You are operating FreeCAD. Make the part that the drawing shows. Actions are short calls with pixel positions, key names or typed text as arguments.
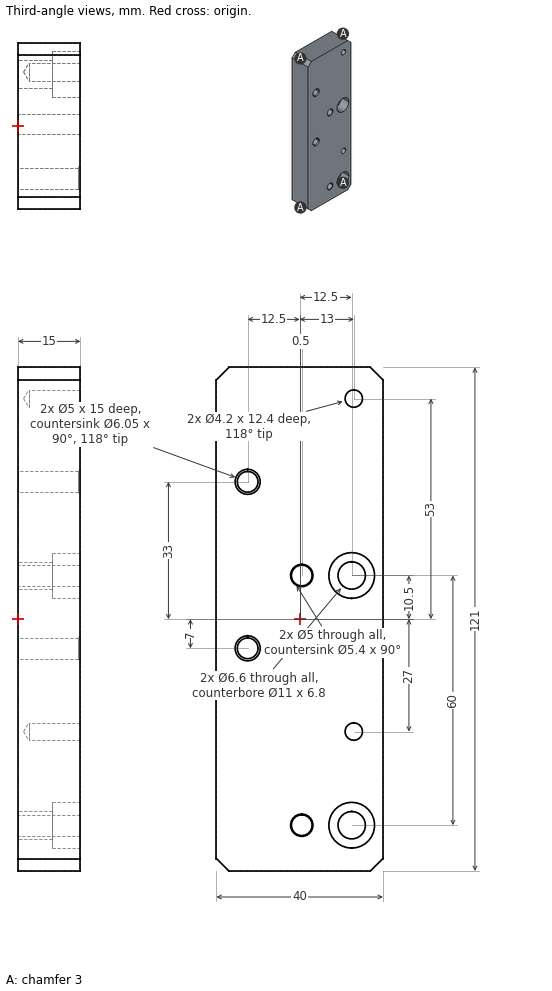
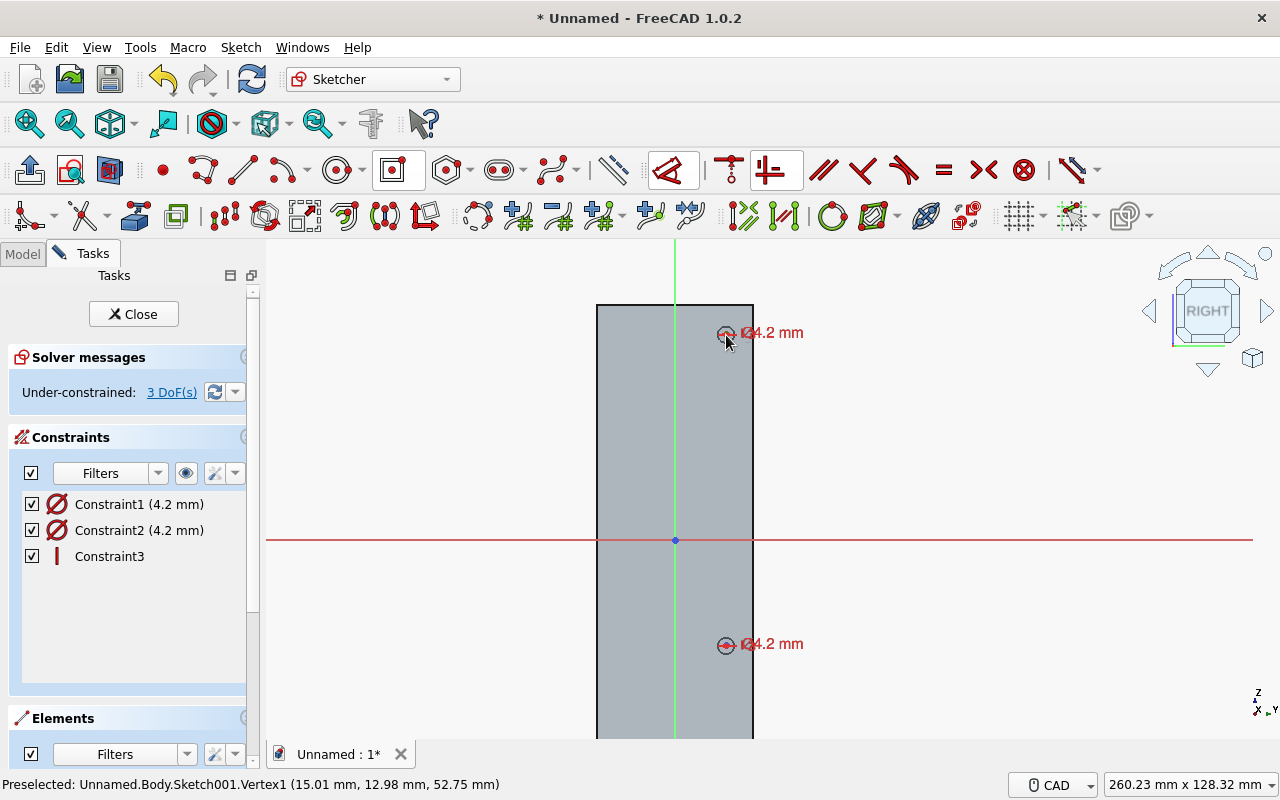
click(694, 170)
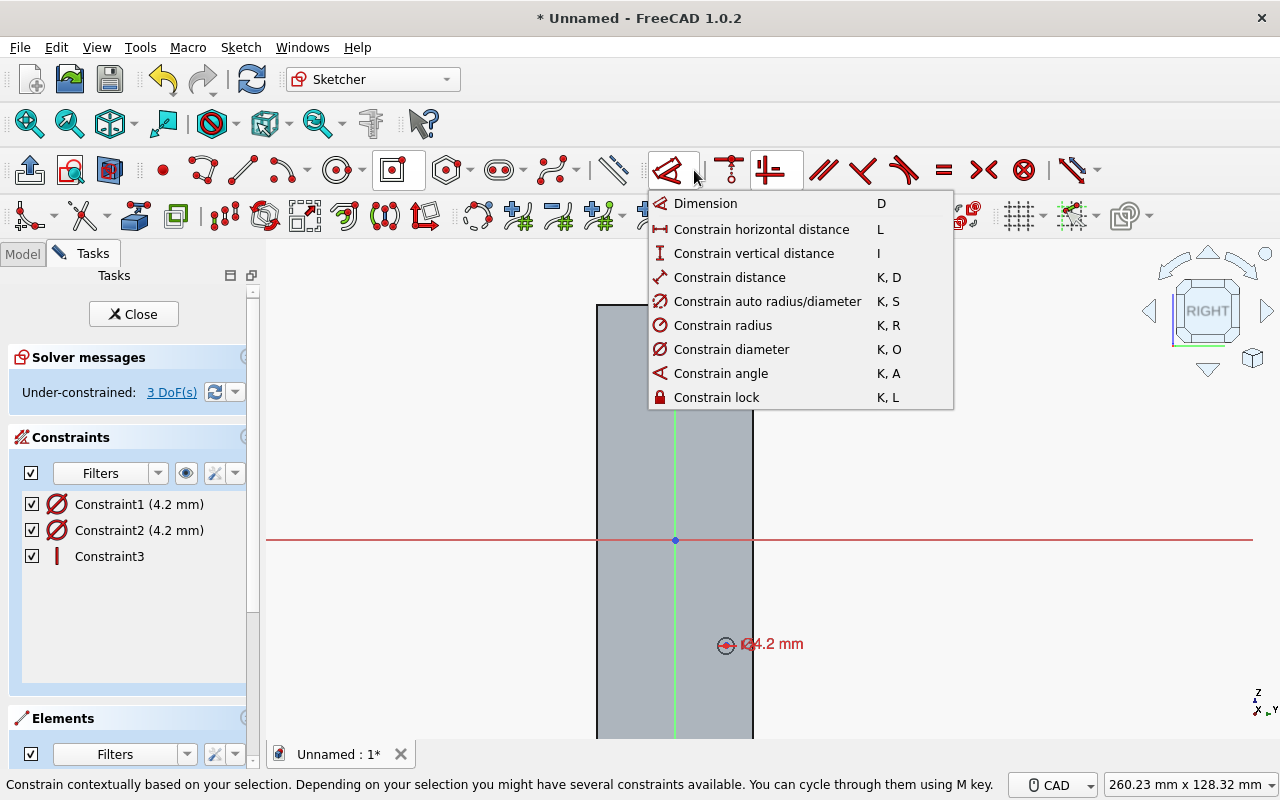
click(801, 229)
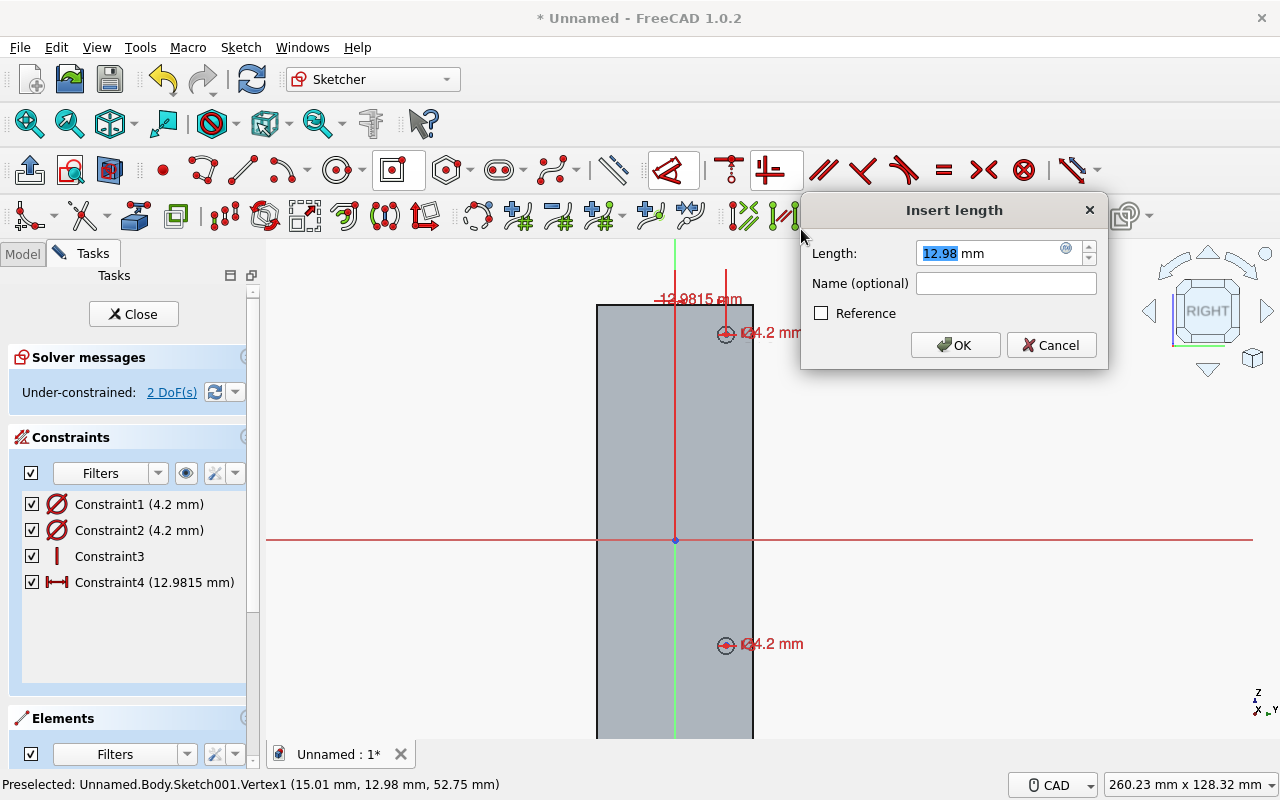
text(13)
key(Return)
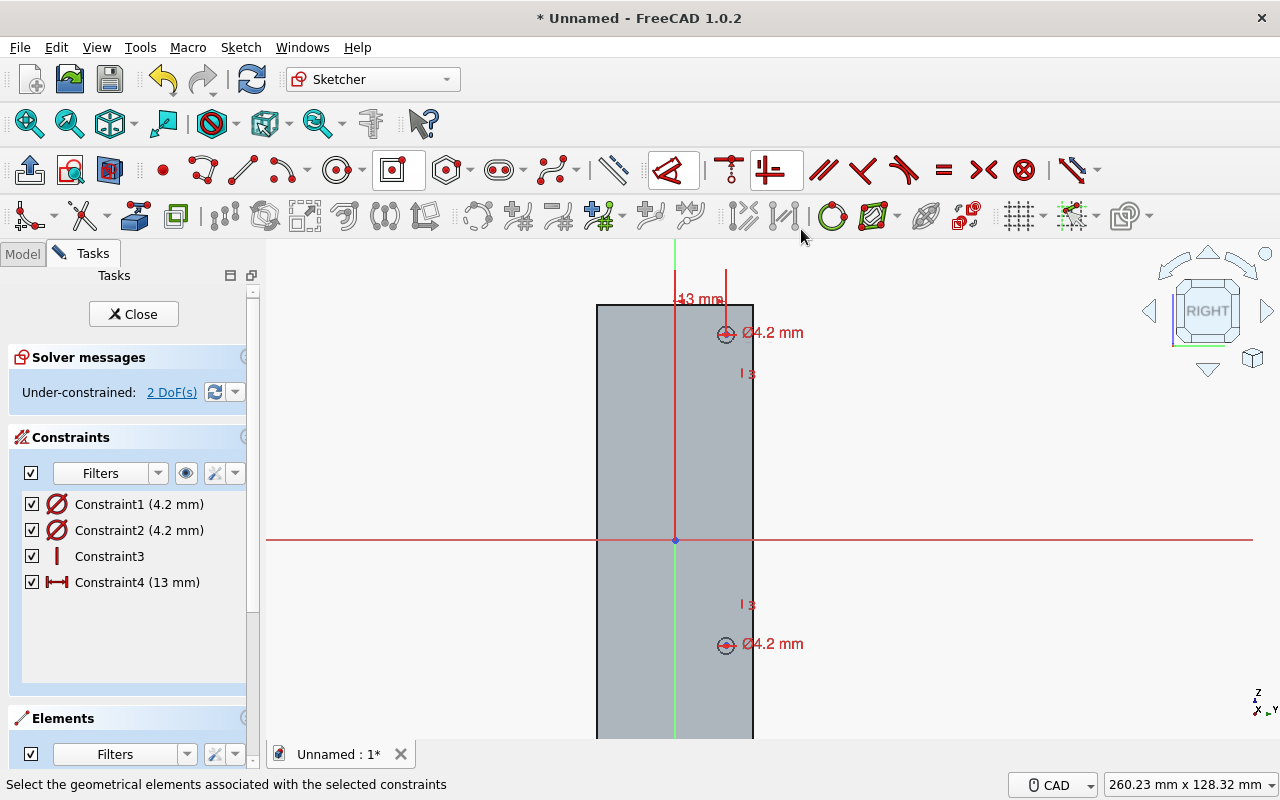
click(726, 335)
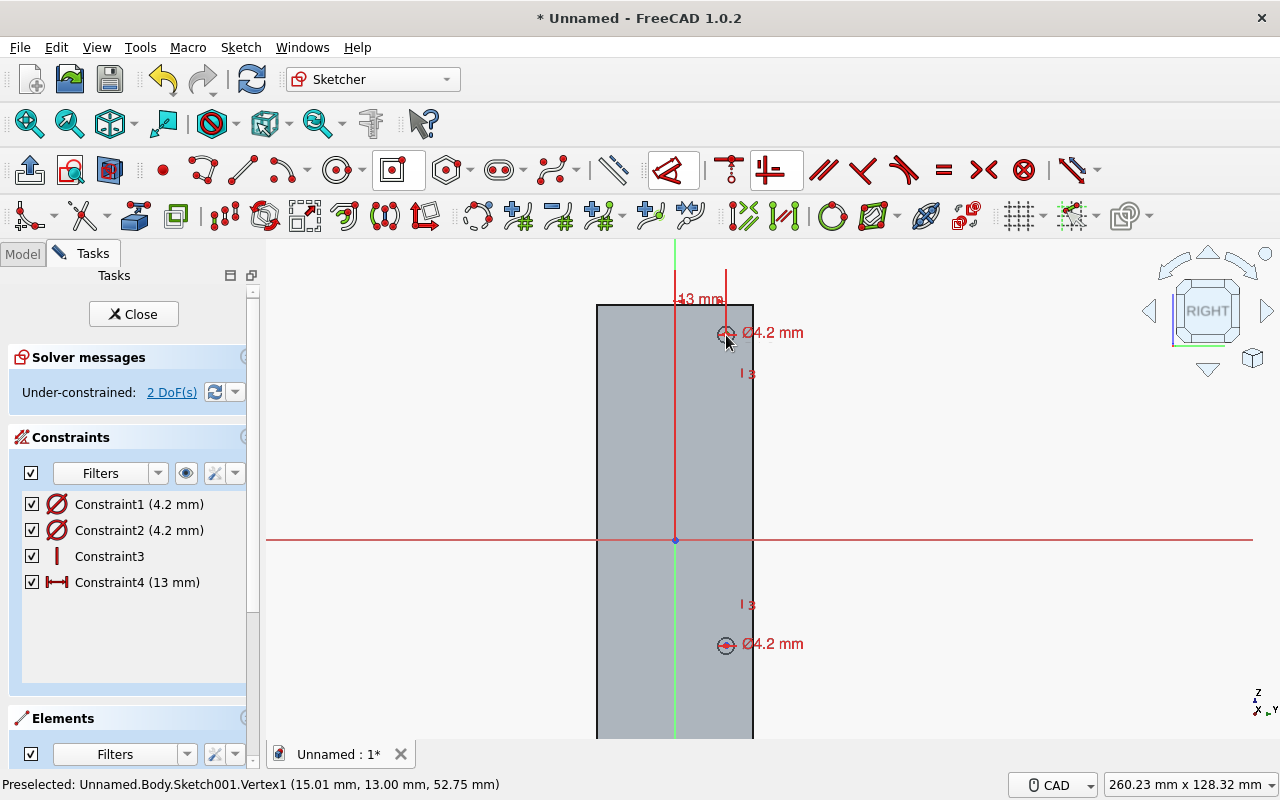
click(694, 170)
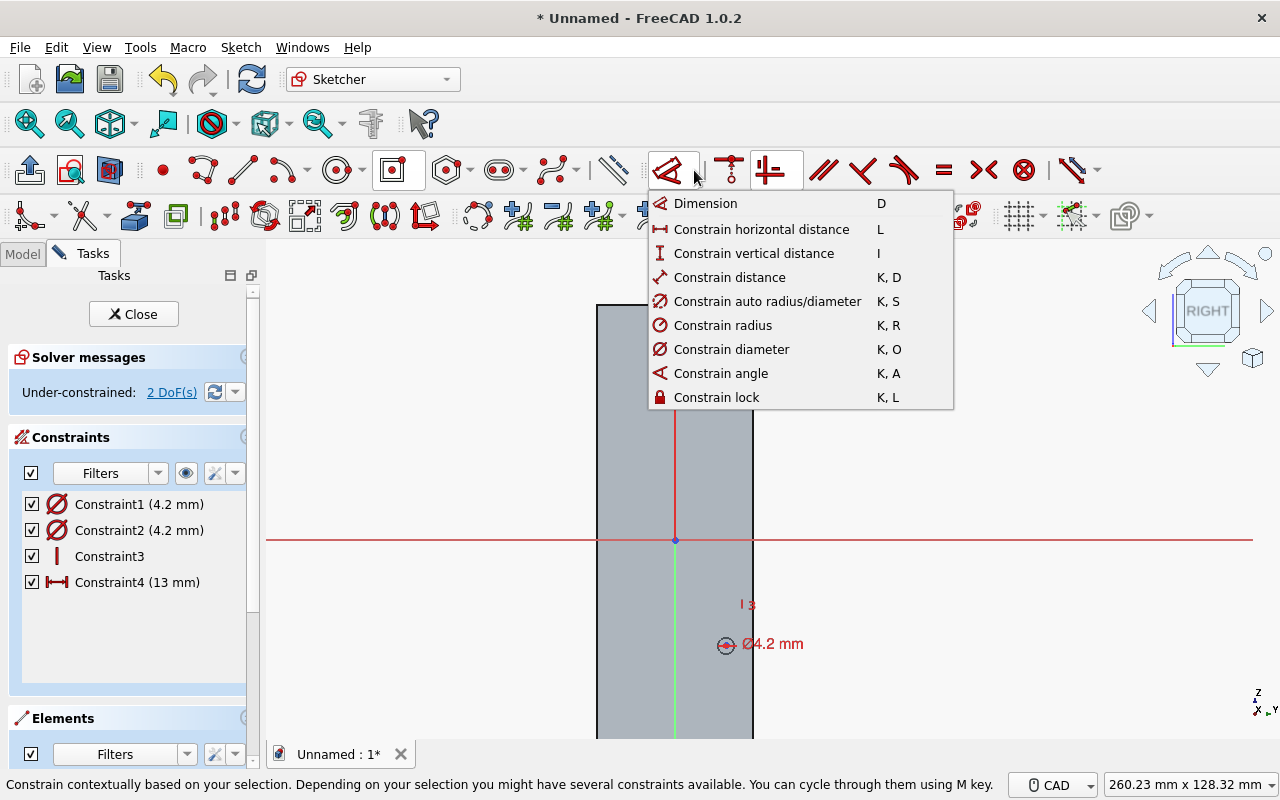
click(801, 253)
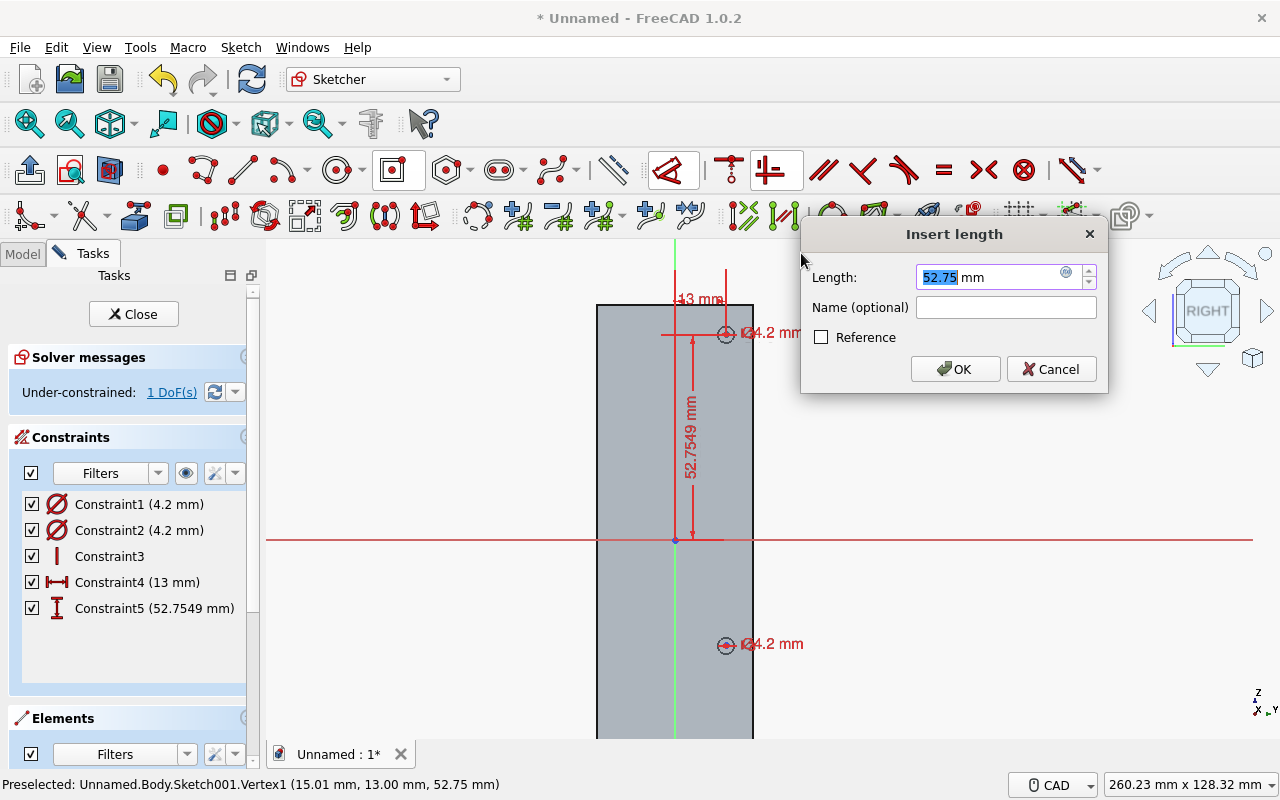
text(53)
key(Return)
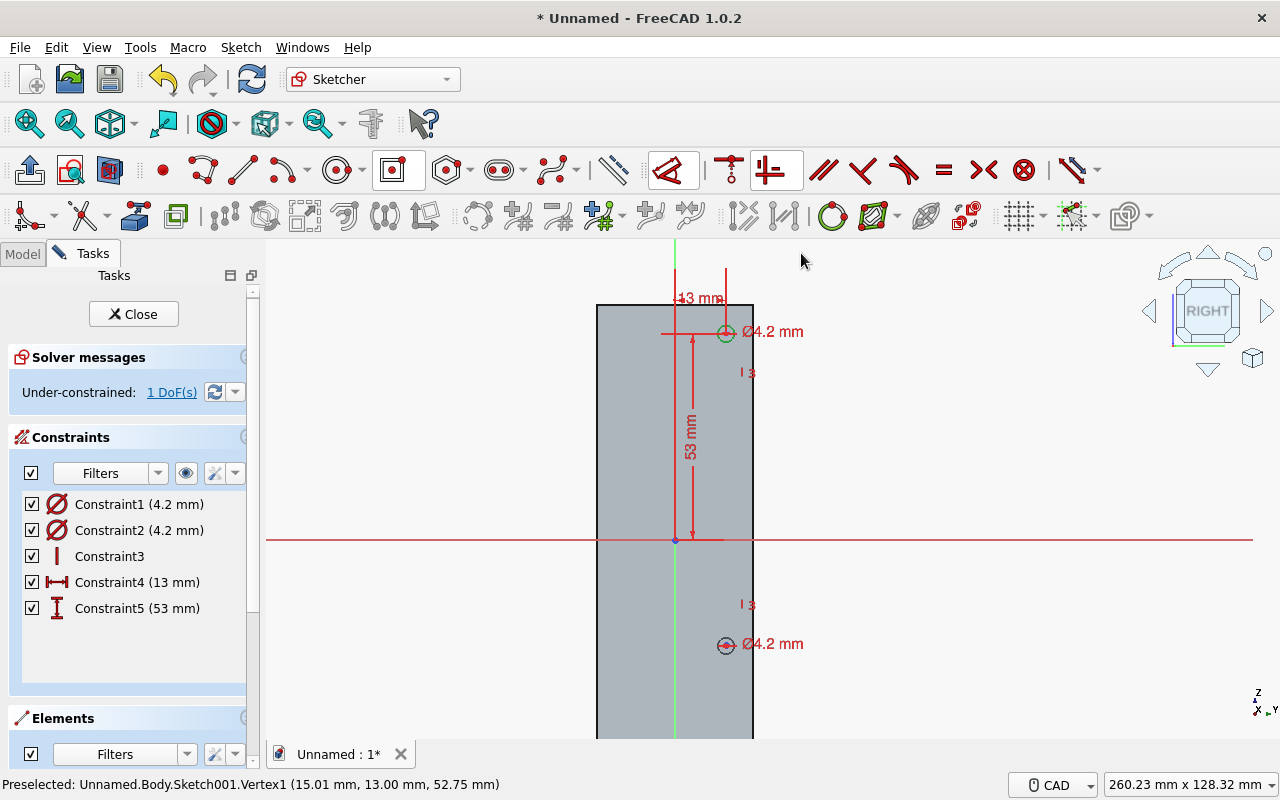
click(726, 646)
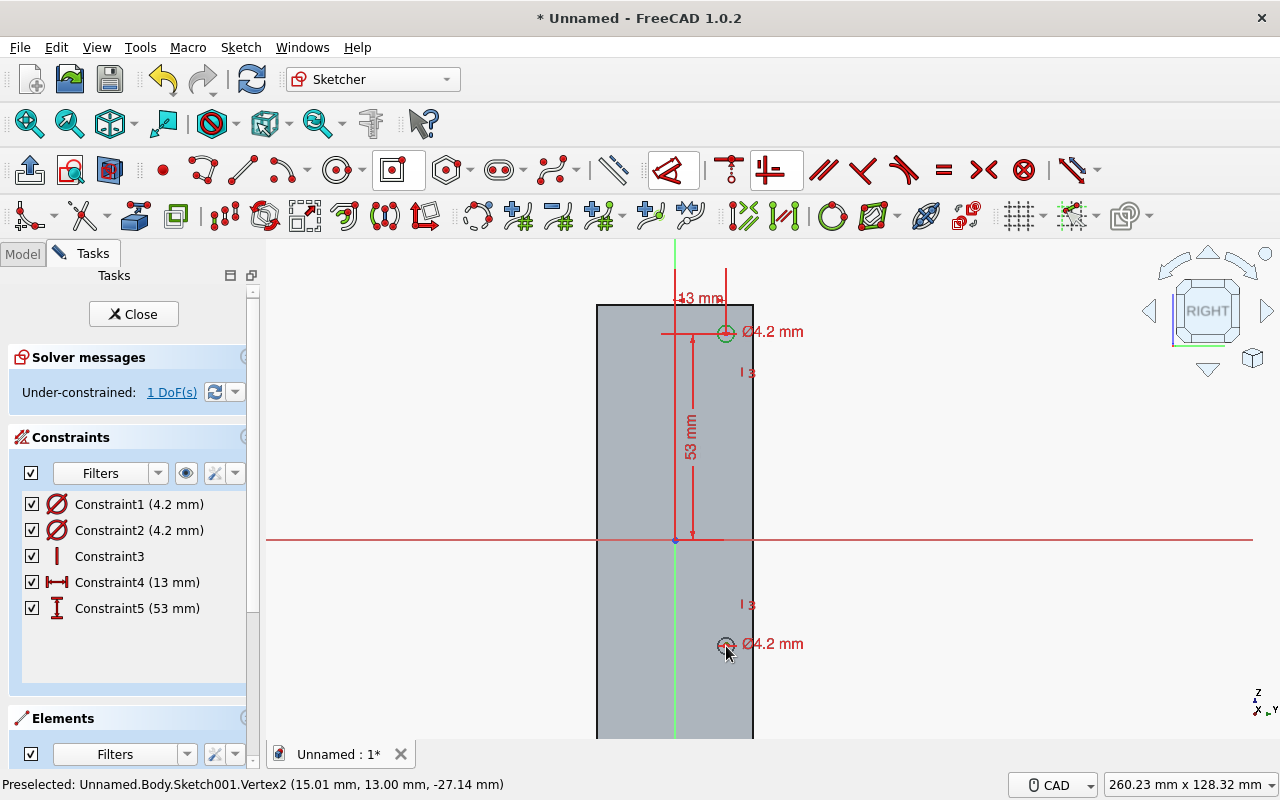
click(694, 170)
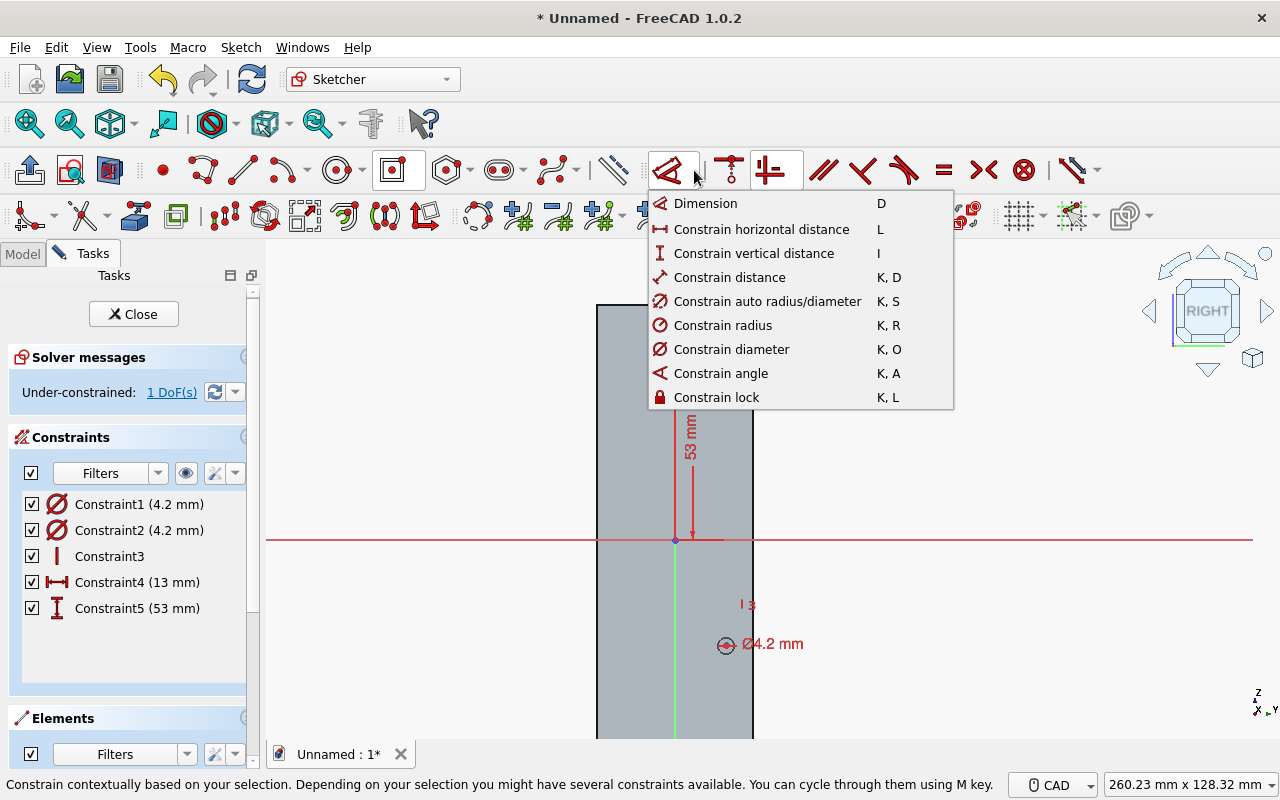
click(801, 253)